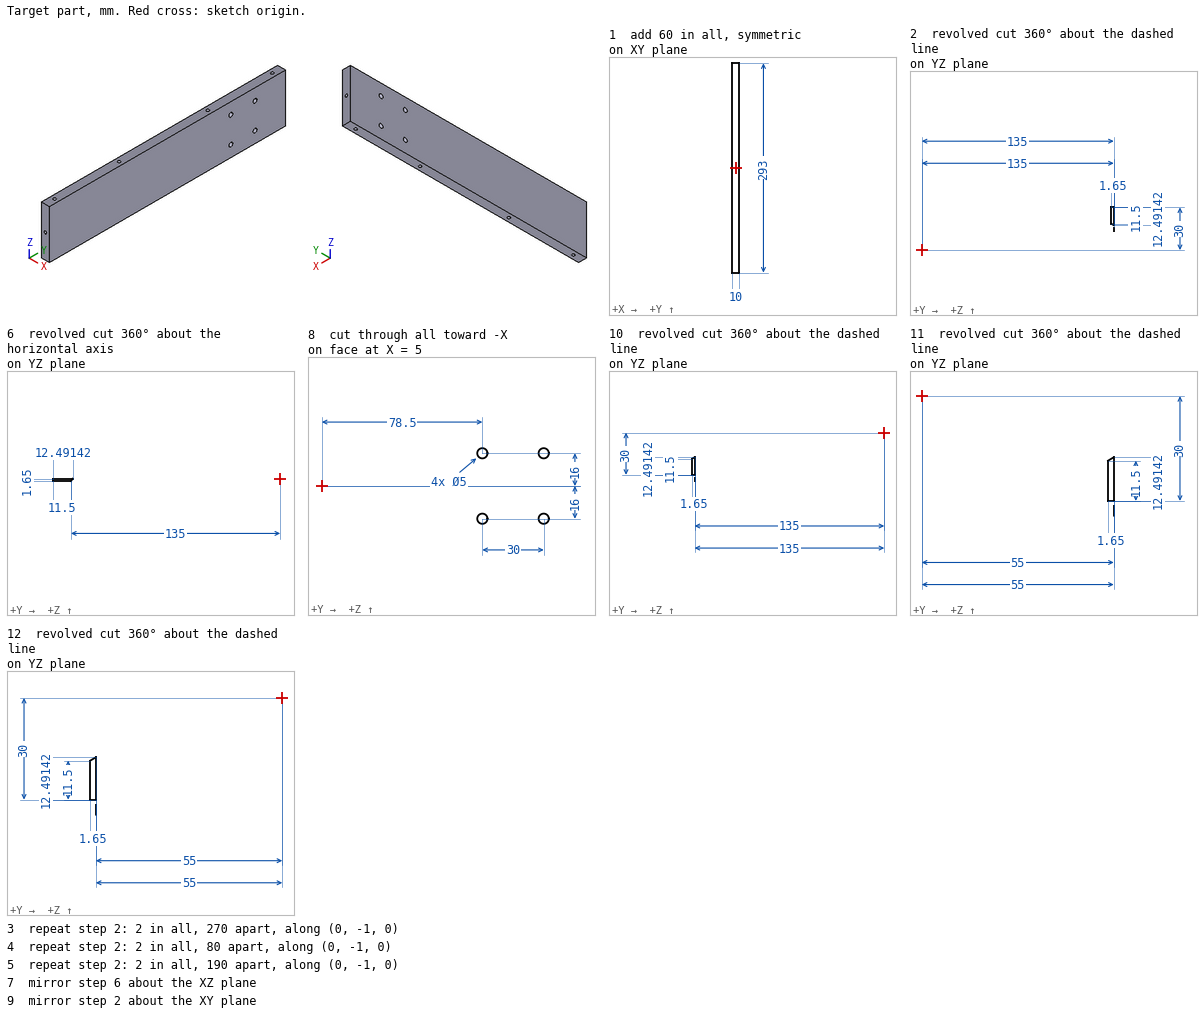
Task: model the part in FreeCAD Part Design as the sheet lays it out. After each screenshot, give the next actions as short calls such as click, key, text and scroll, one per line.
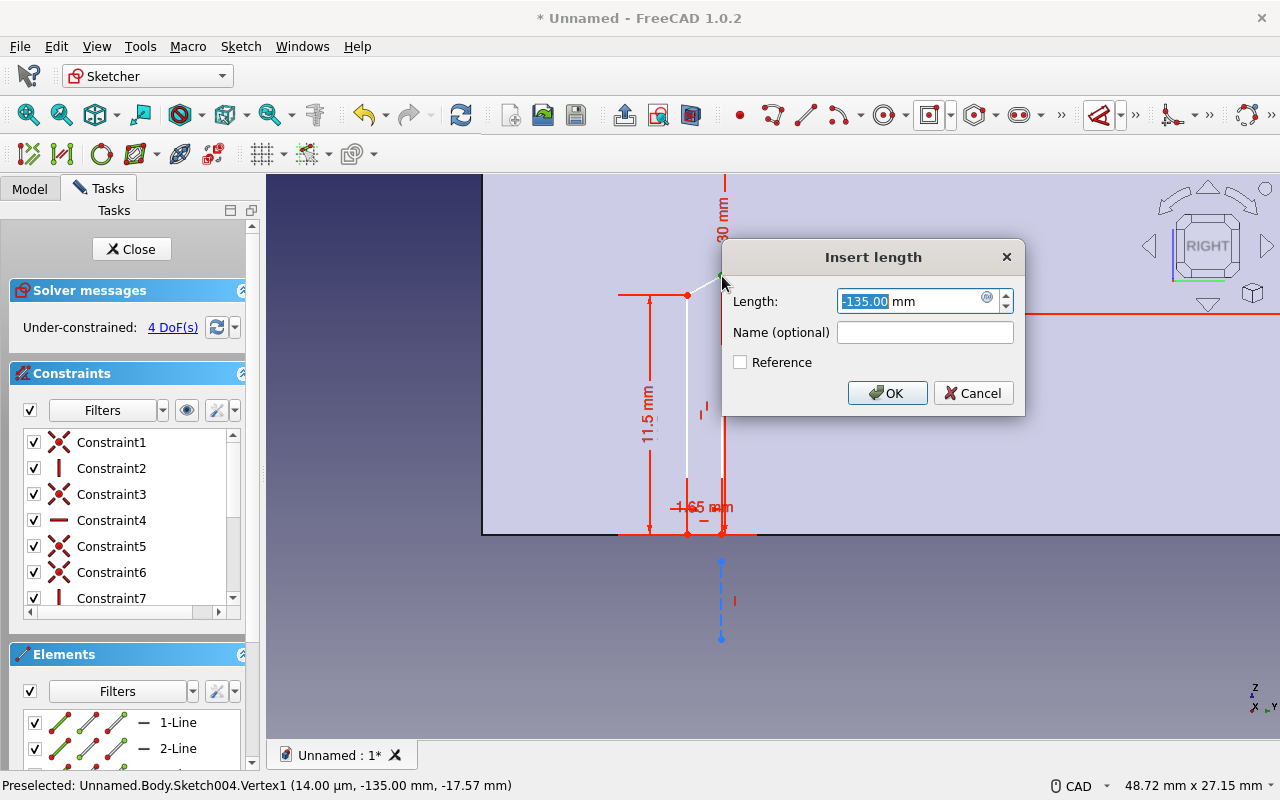
text(-135)
key(Return)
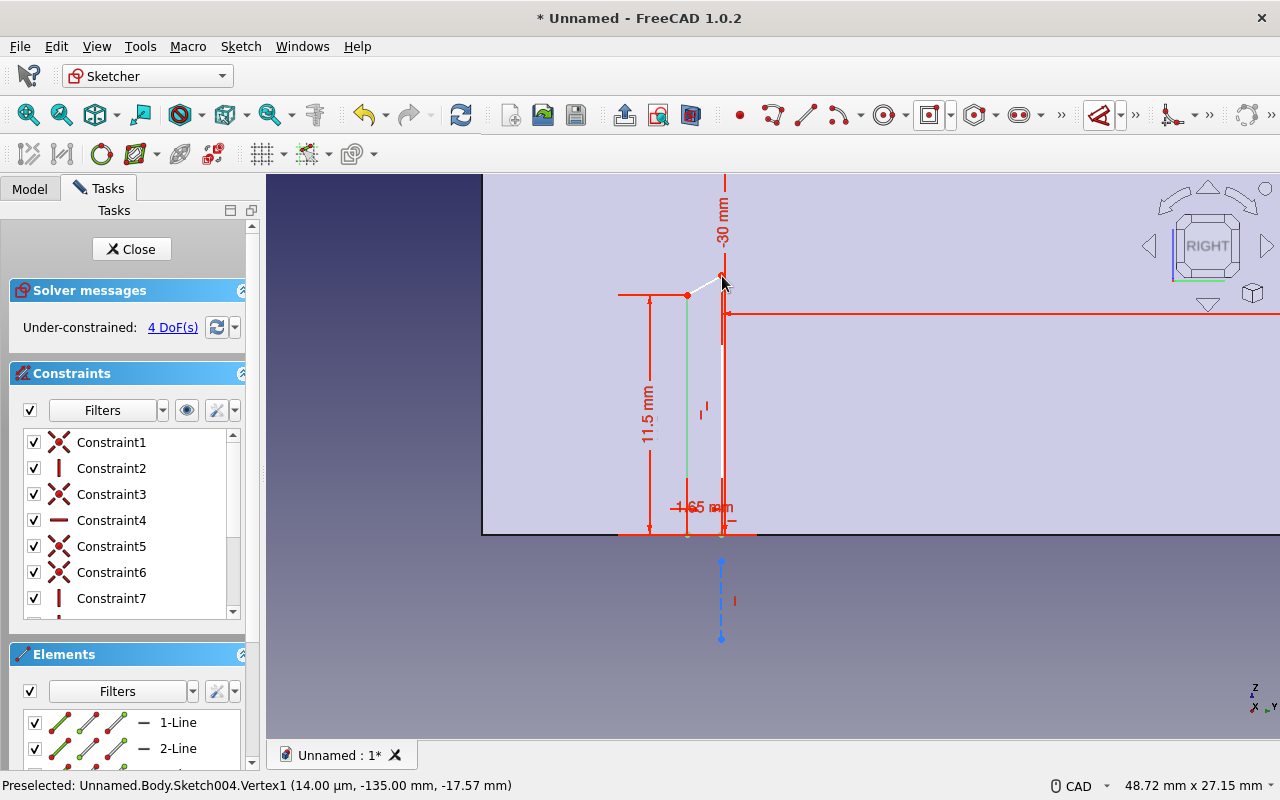
click(721, 562)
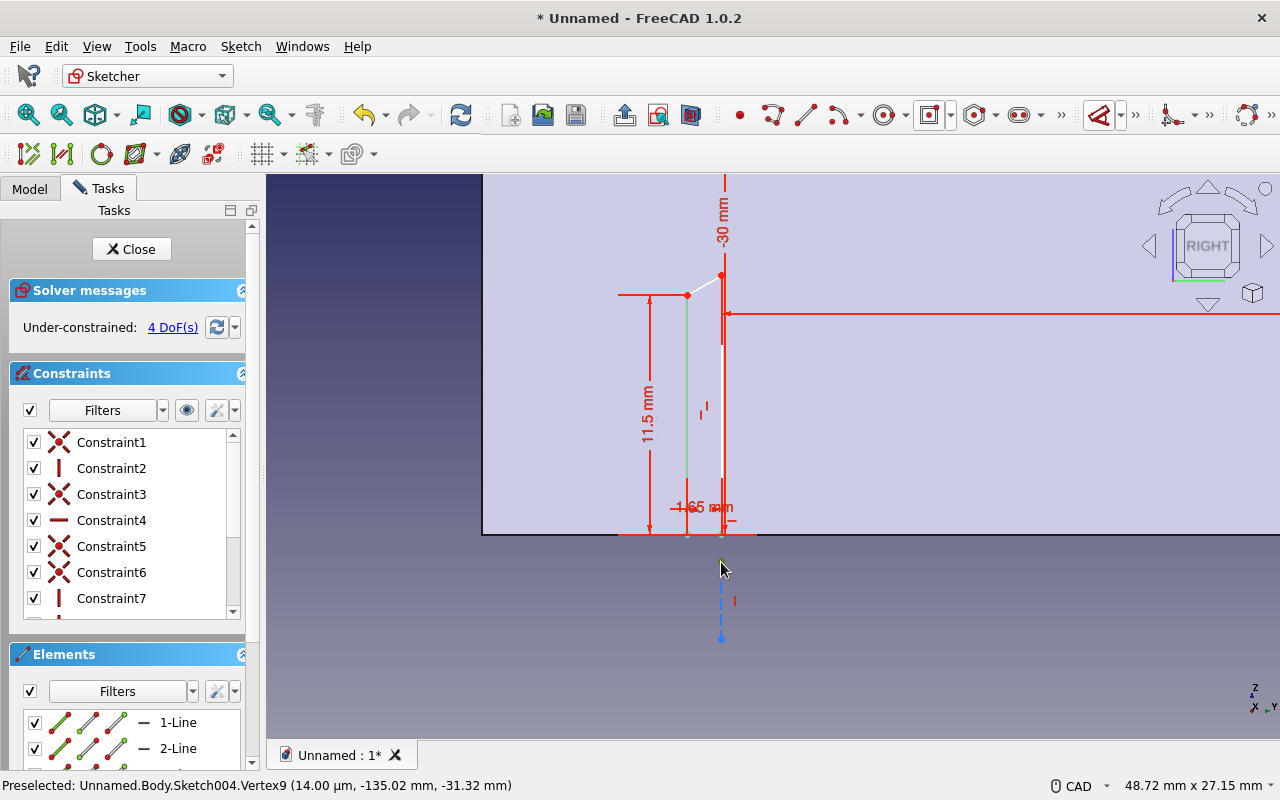
key(l)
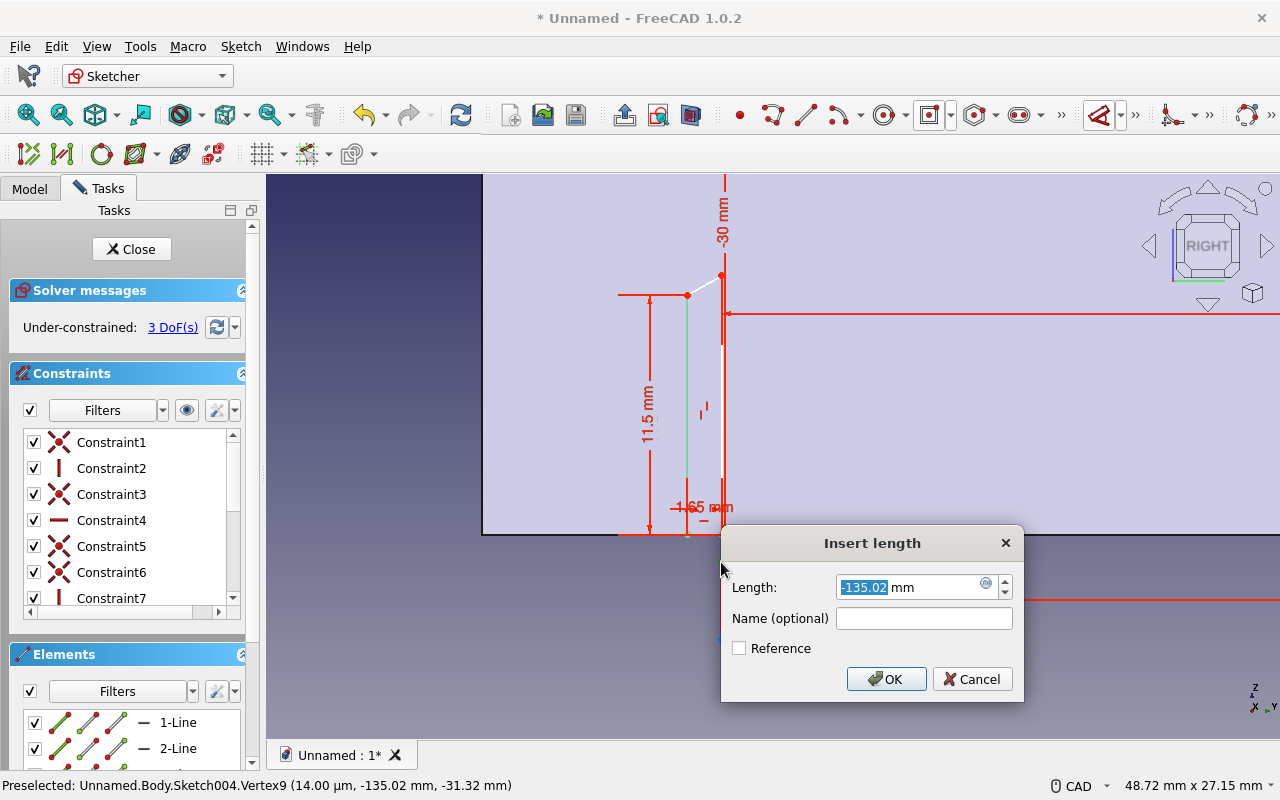
text(-135)
key(Return)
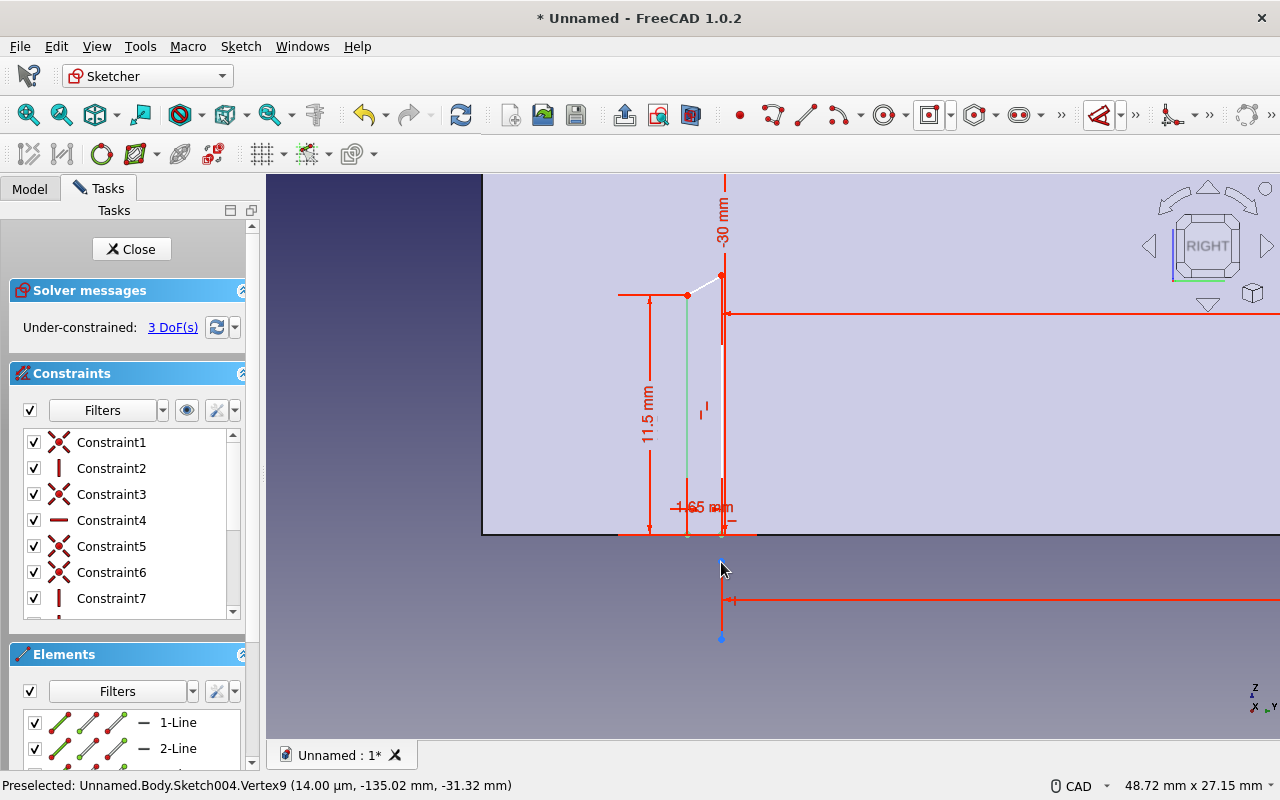
click(722, 457)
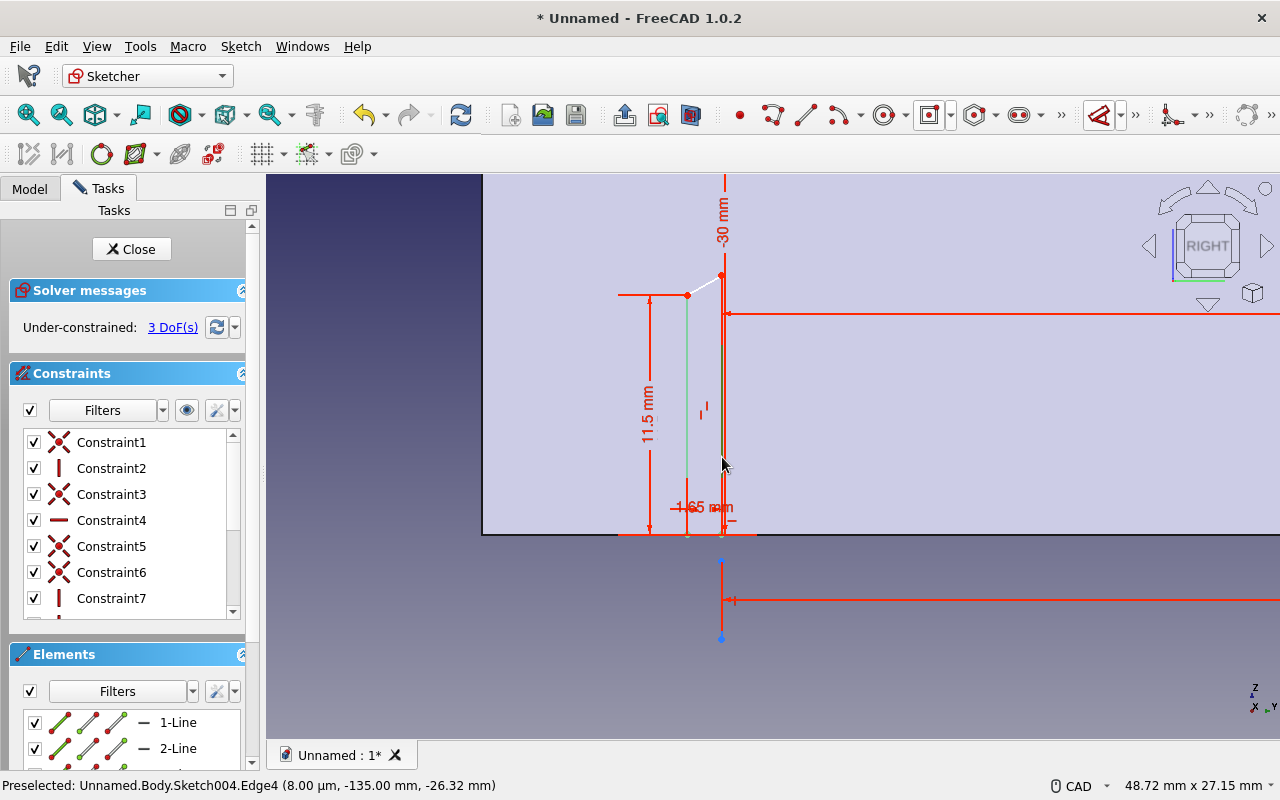
key(i)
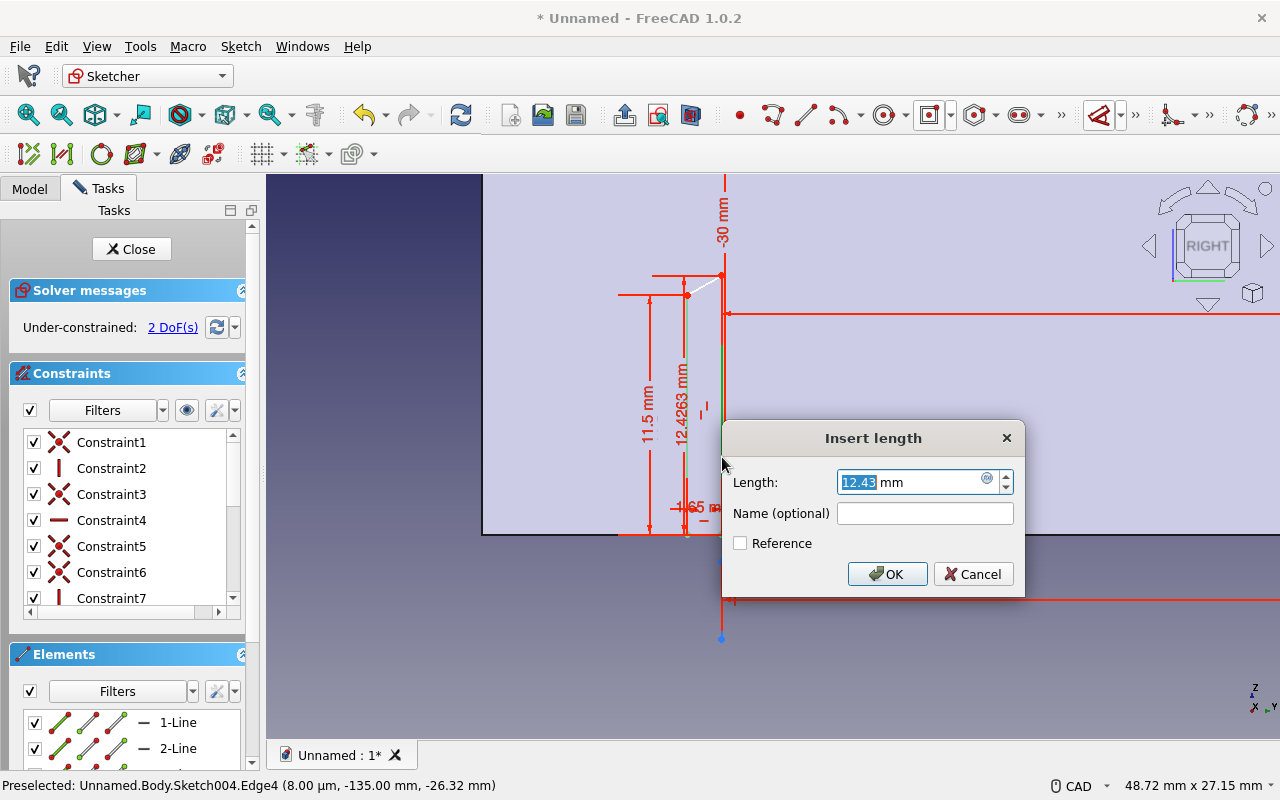
text(12.49142)
key(Return)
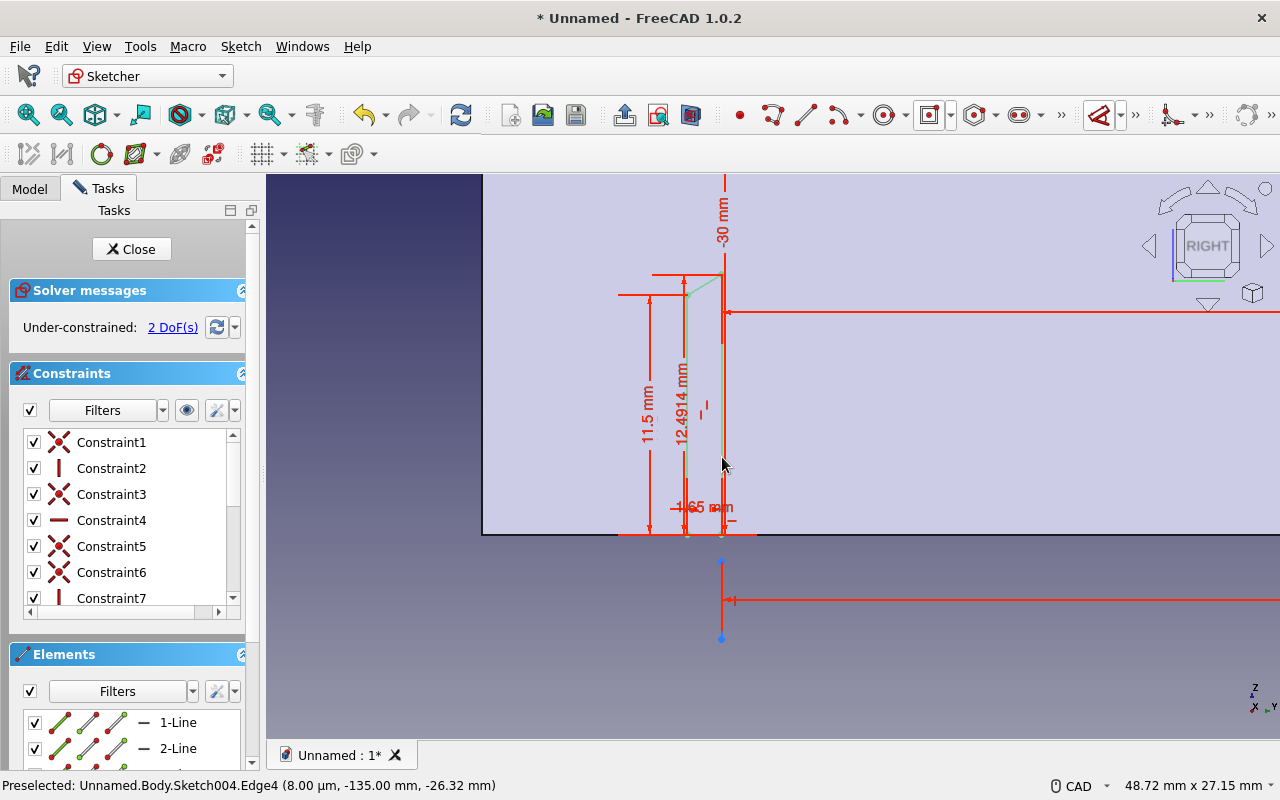
click(132, 249)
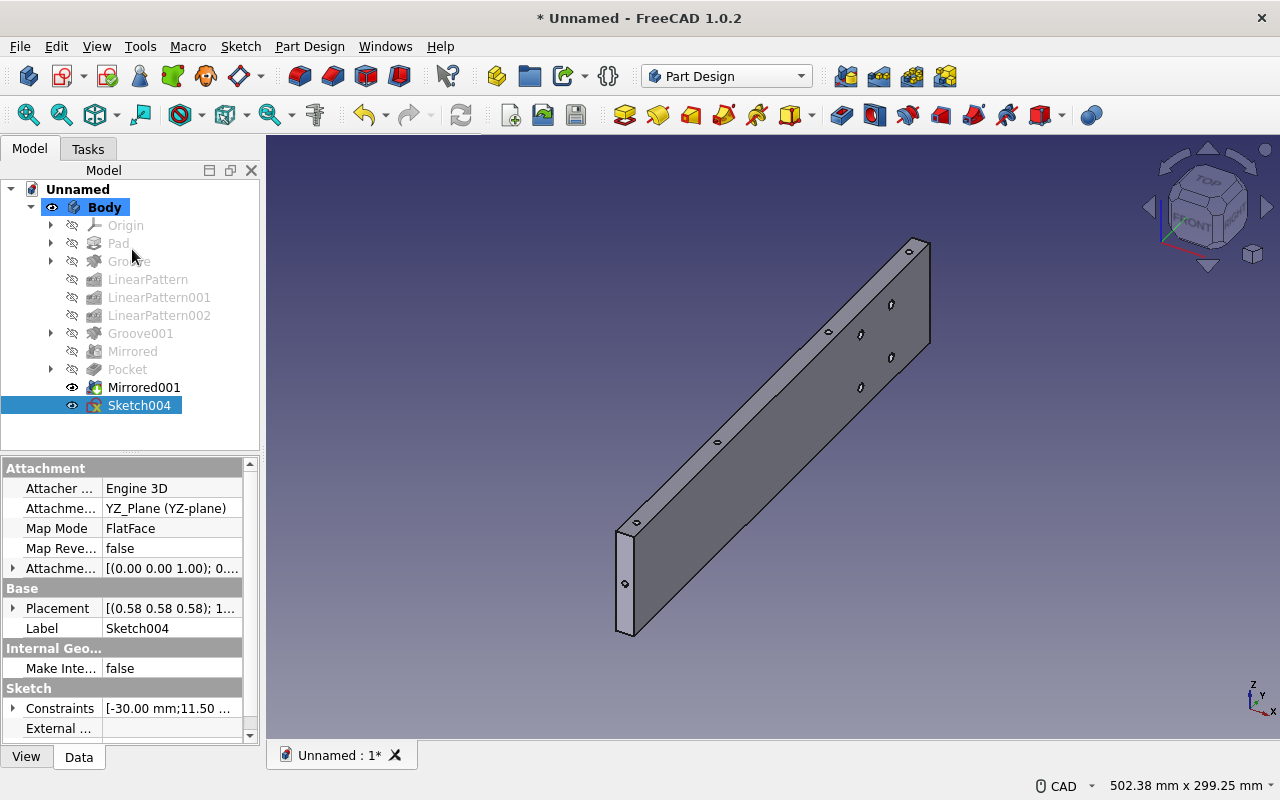
click(908, 116)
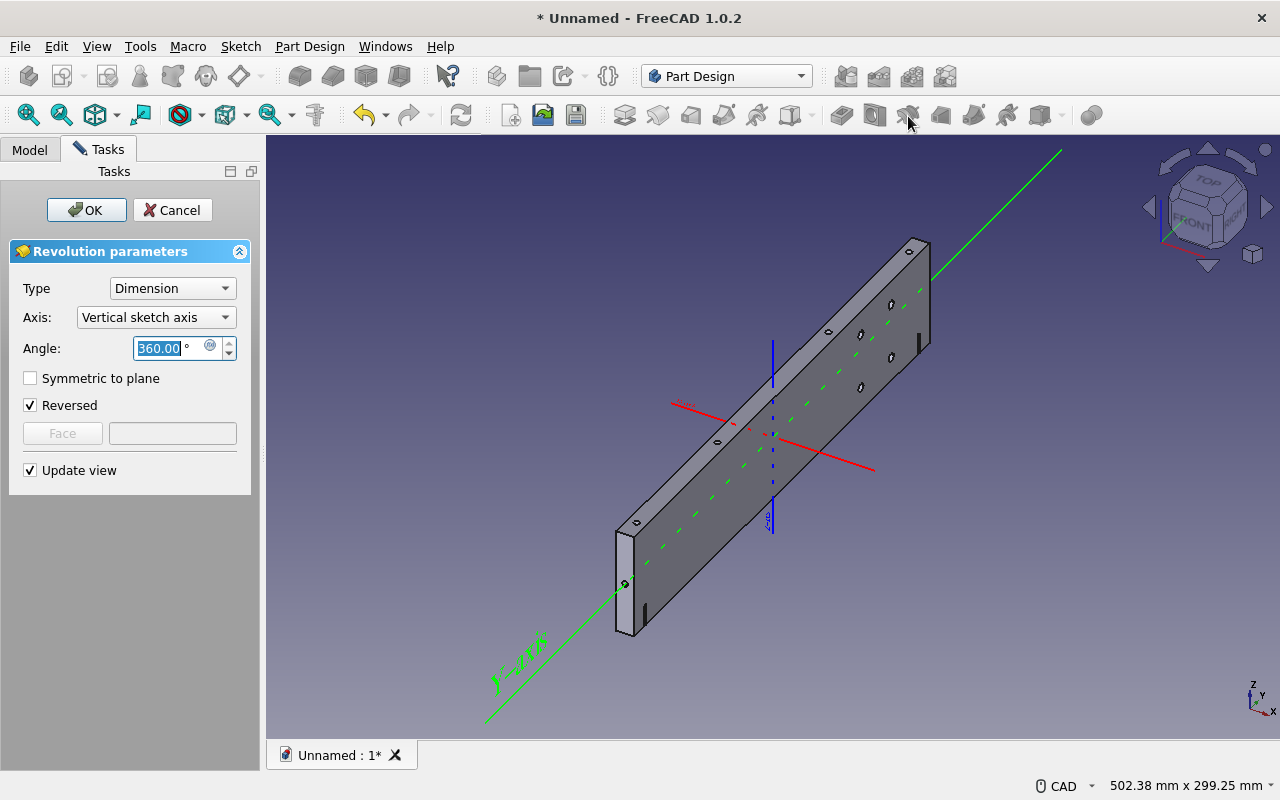
click(157, 318)